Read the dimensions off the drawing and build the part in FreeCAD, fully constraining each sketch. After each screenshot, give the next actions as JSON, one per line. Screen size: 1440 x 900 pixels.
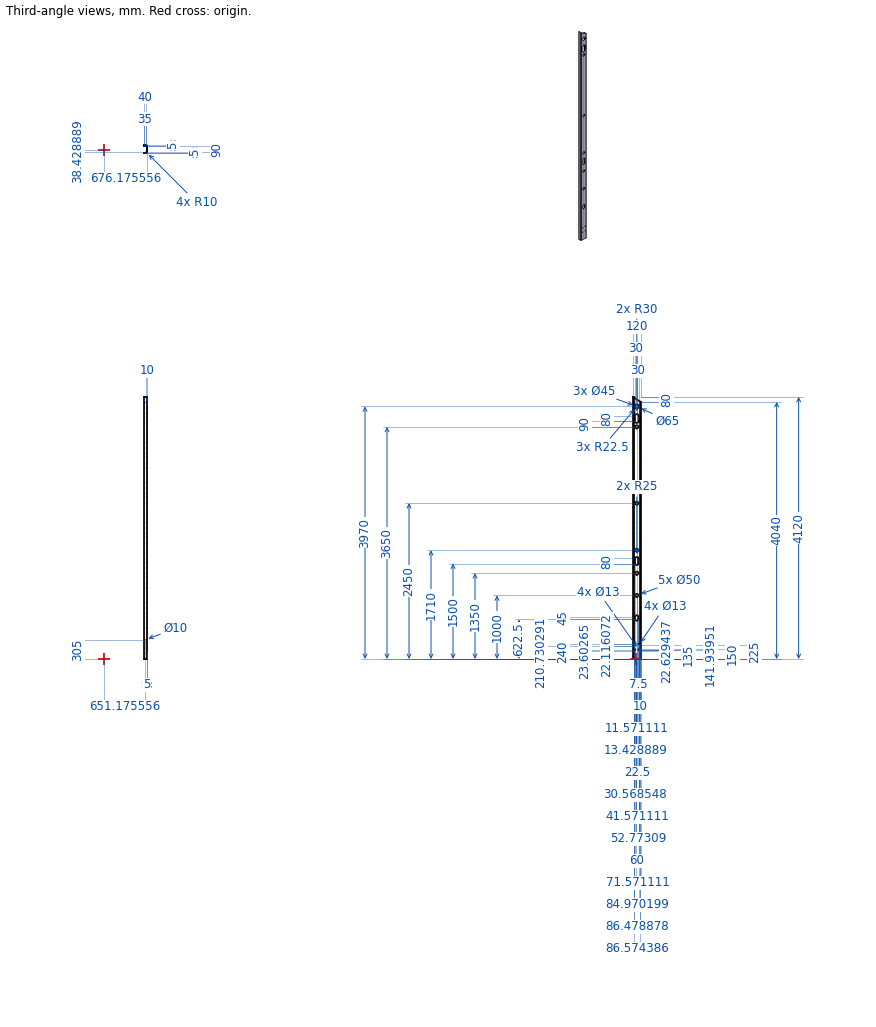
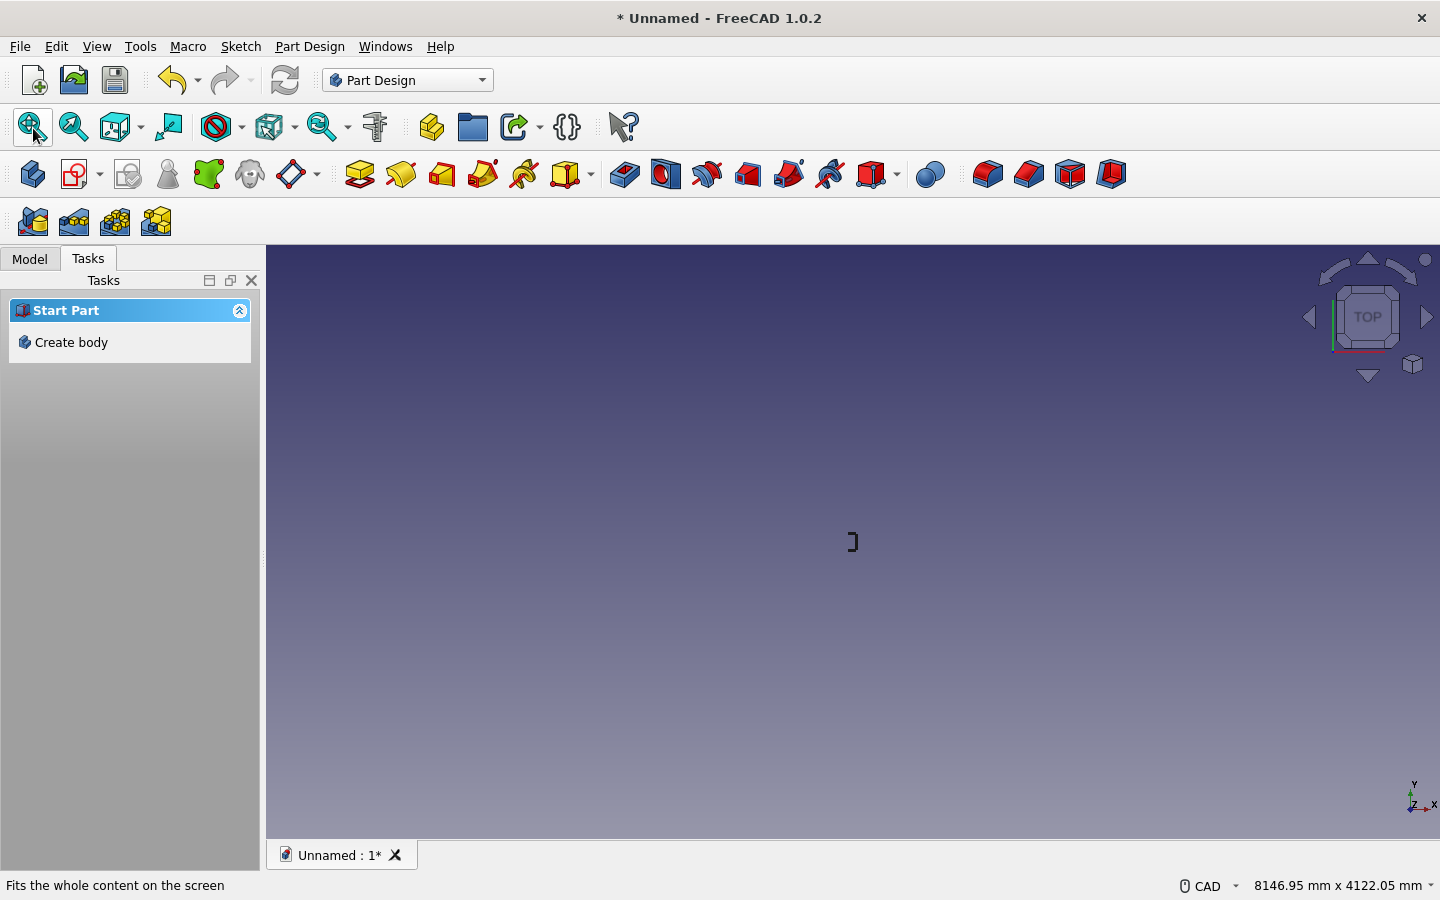
{"action": "key", "text": "v f"}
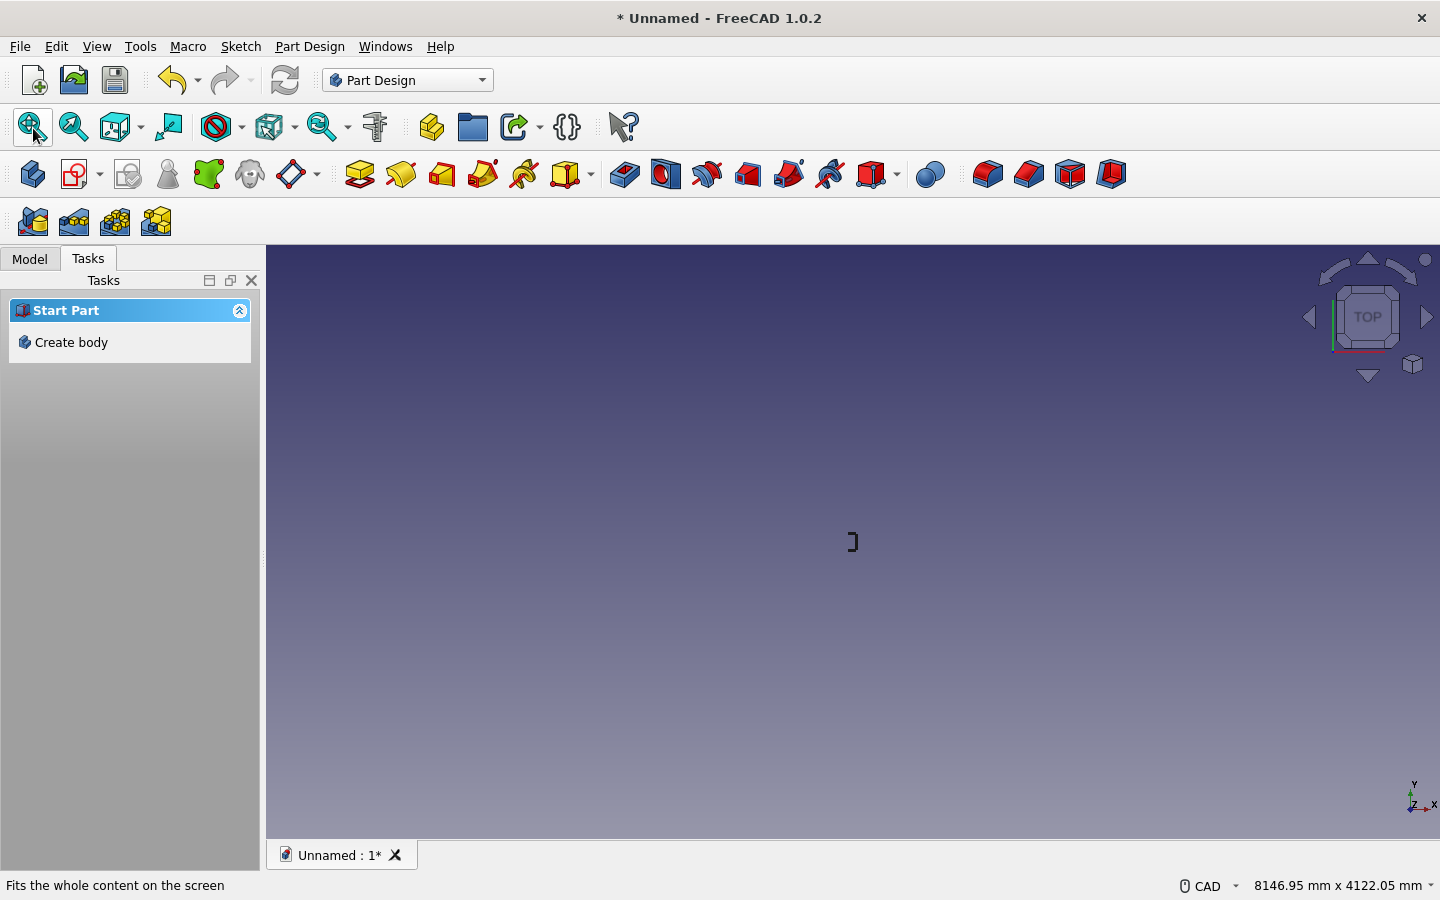
{"action": "left_click", "coordinate": [30, 258]}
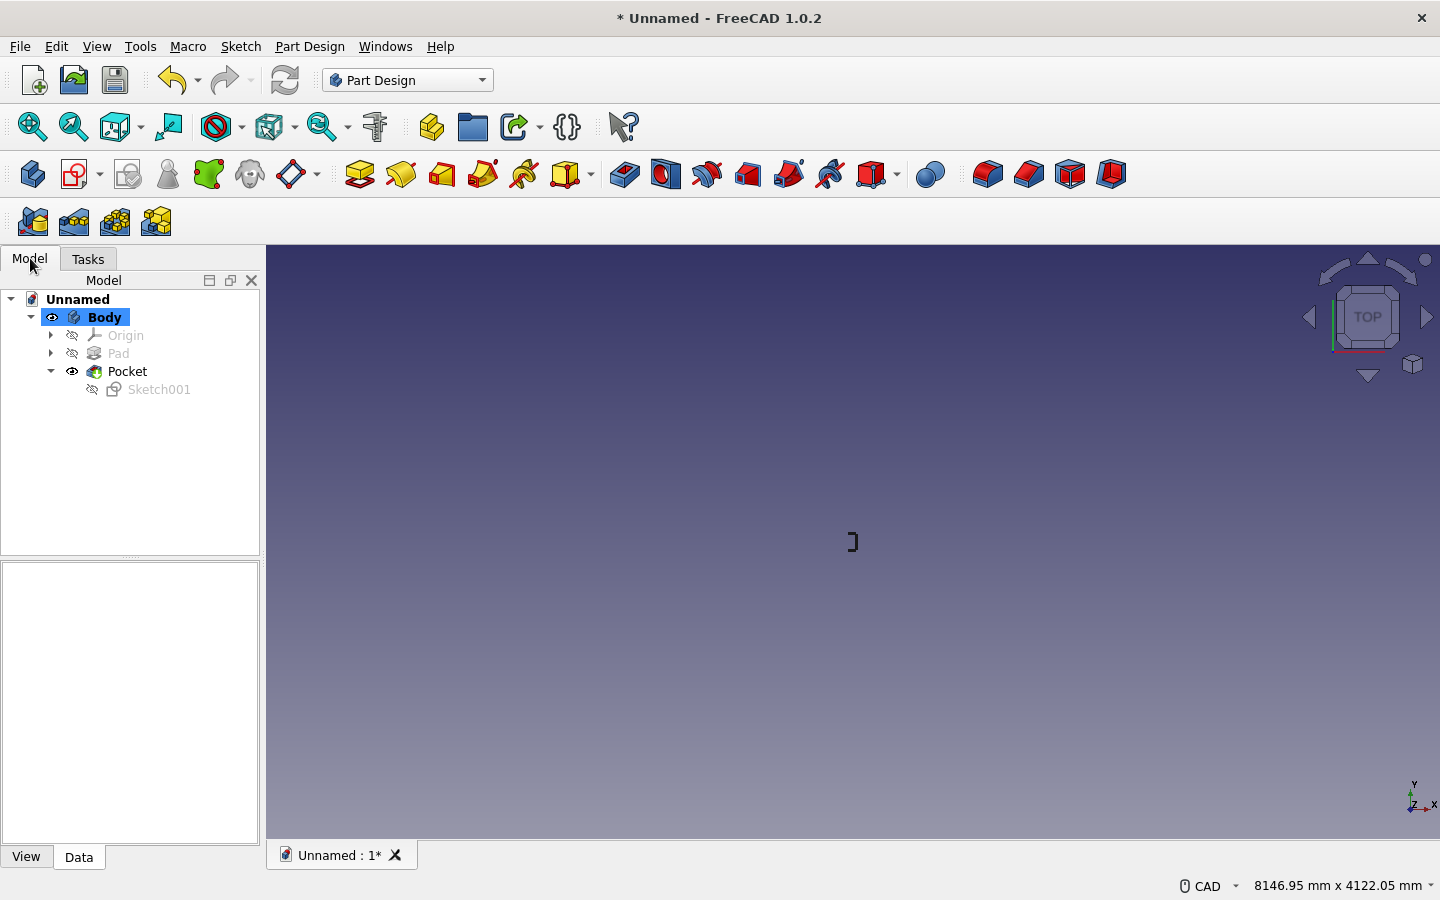
{"action": "left_click", "coordinate": [51, 335]}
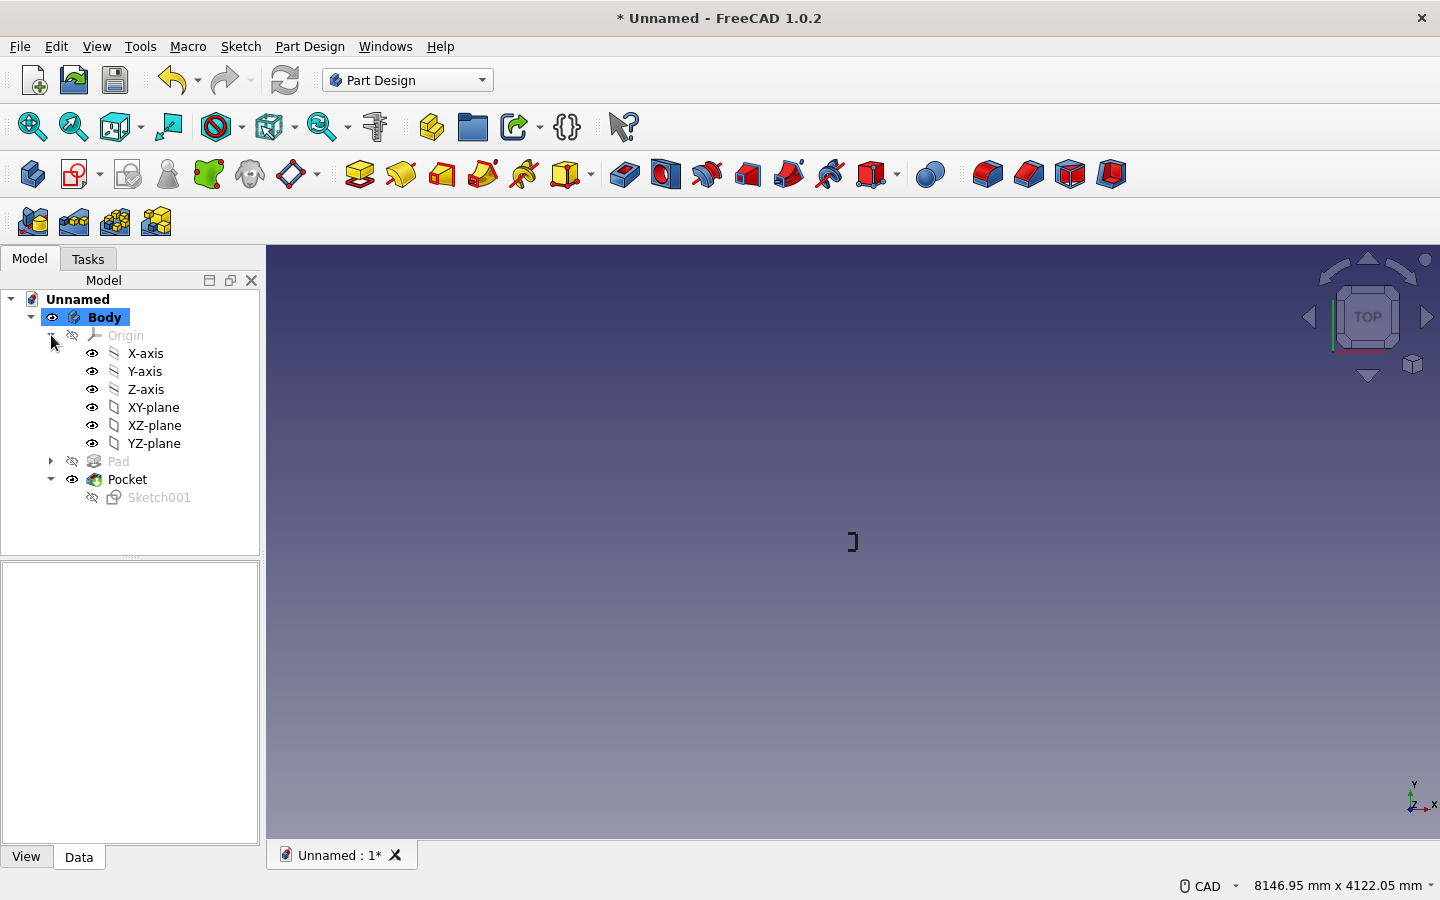
{"action": "left_click", "coordinate": [137, 443]}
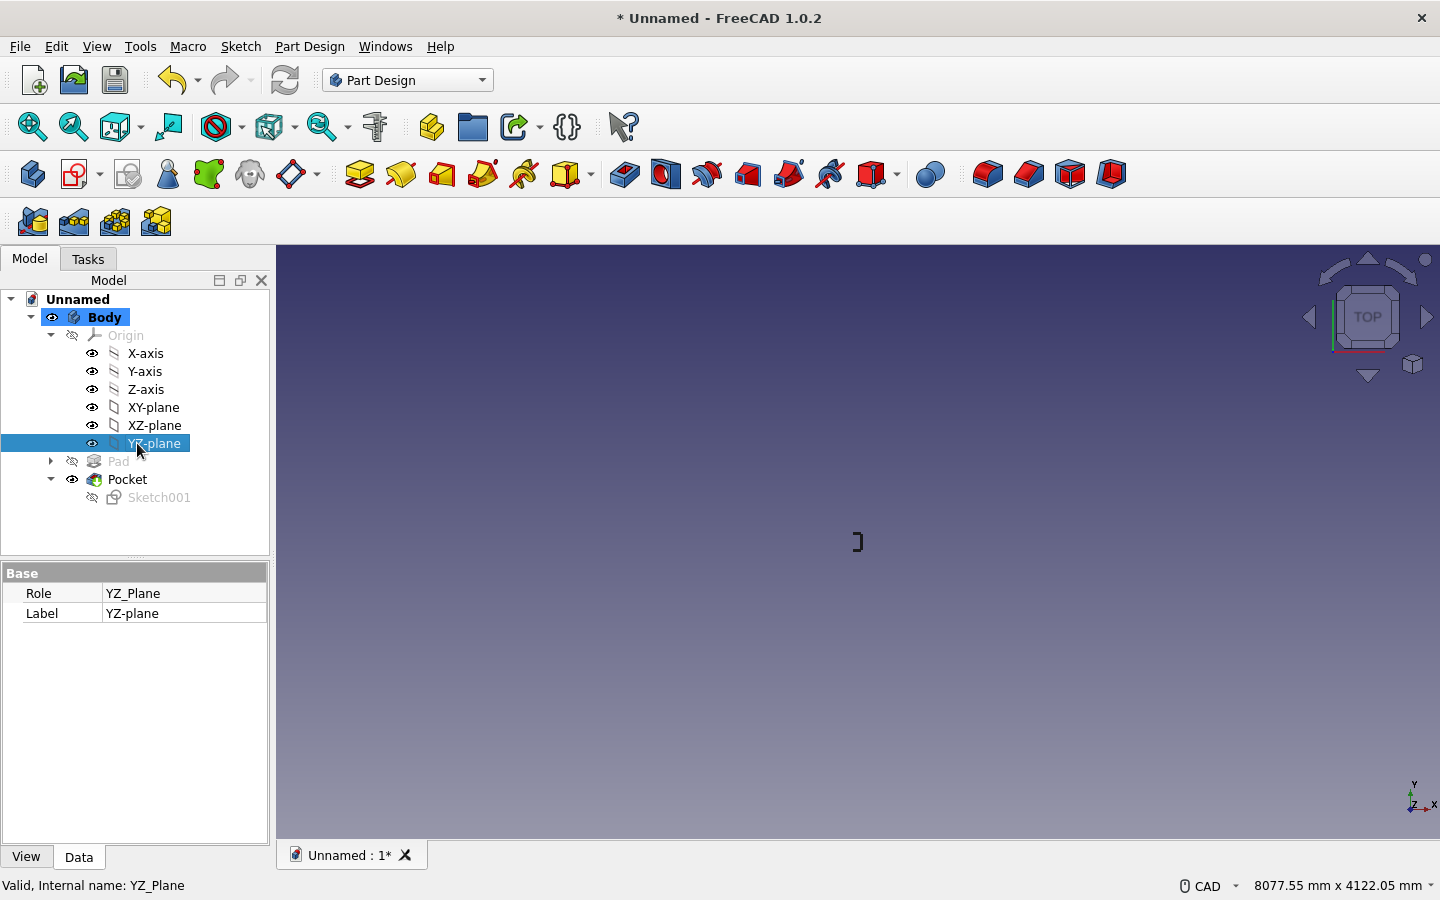
{"action": "left_click", "coordinate": [290, 174]}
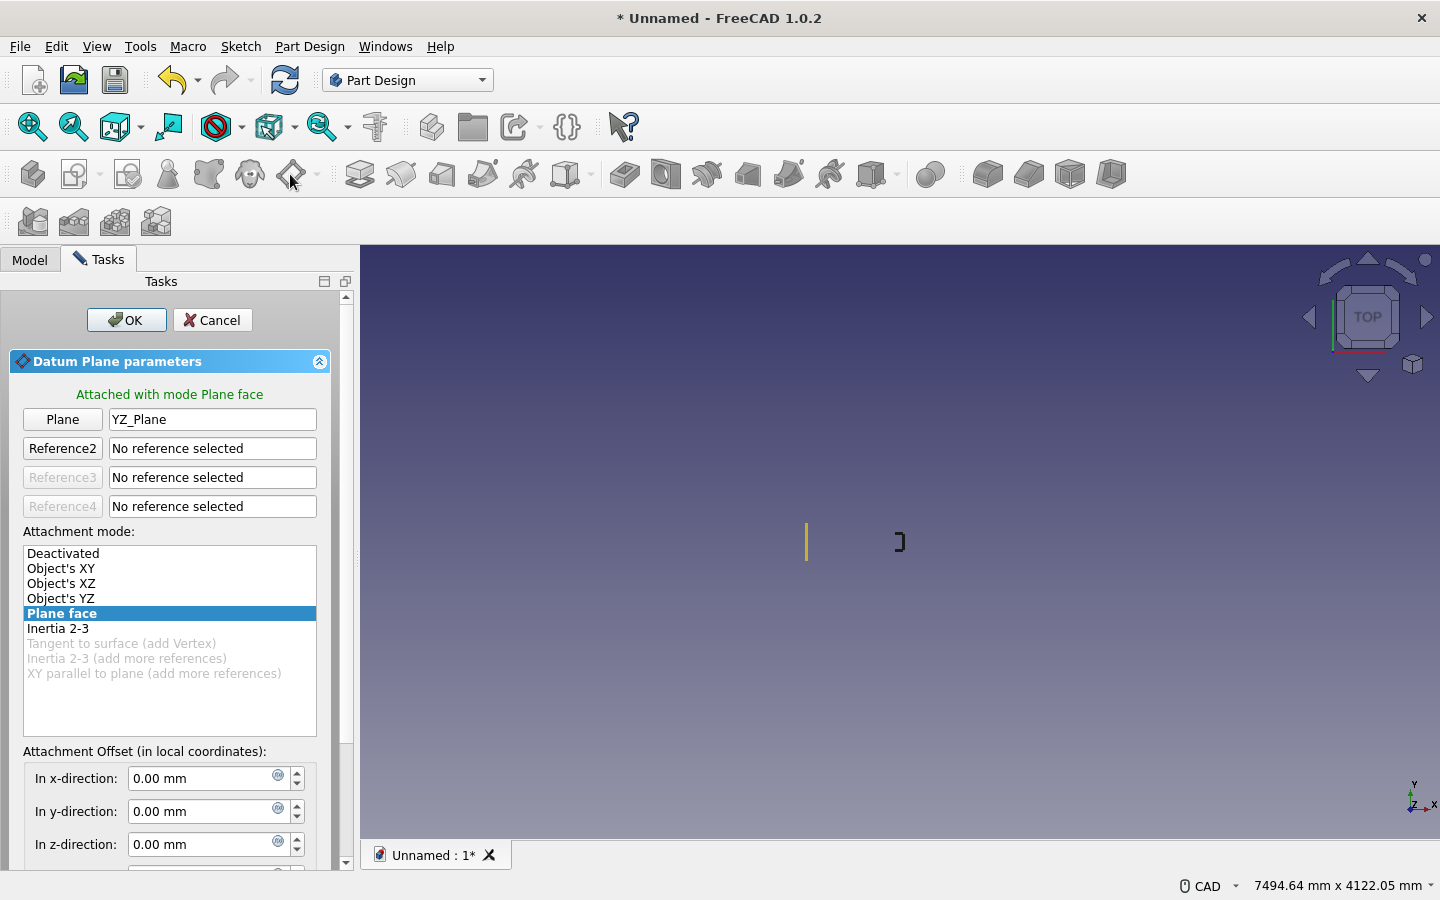
{"action": "triple_click", "coordinate": [210, 844]}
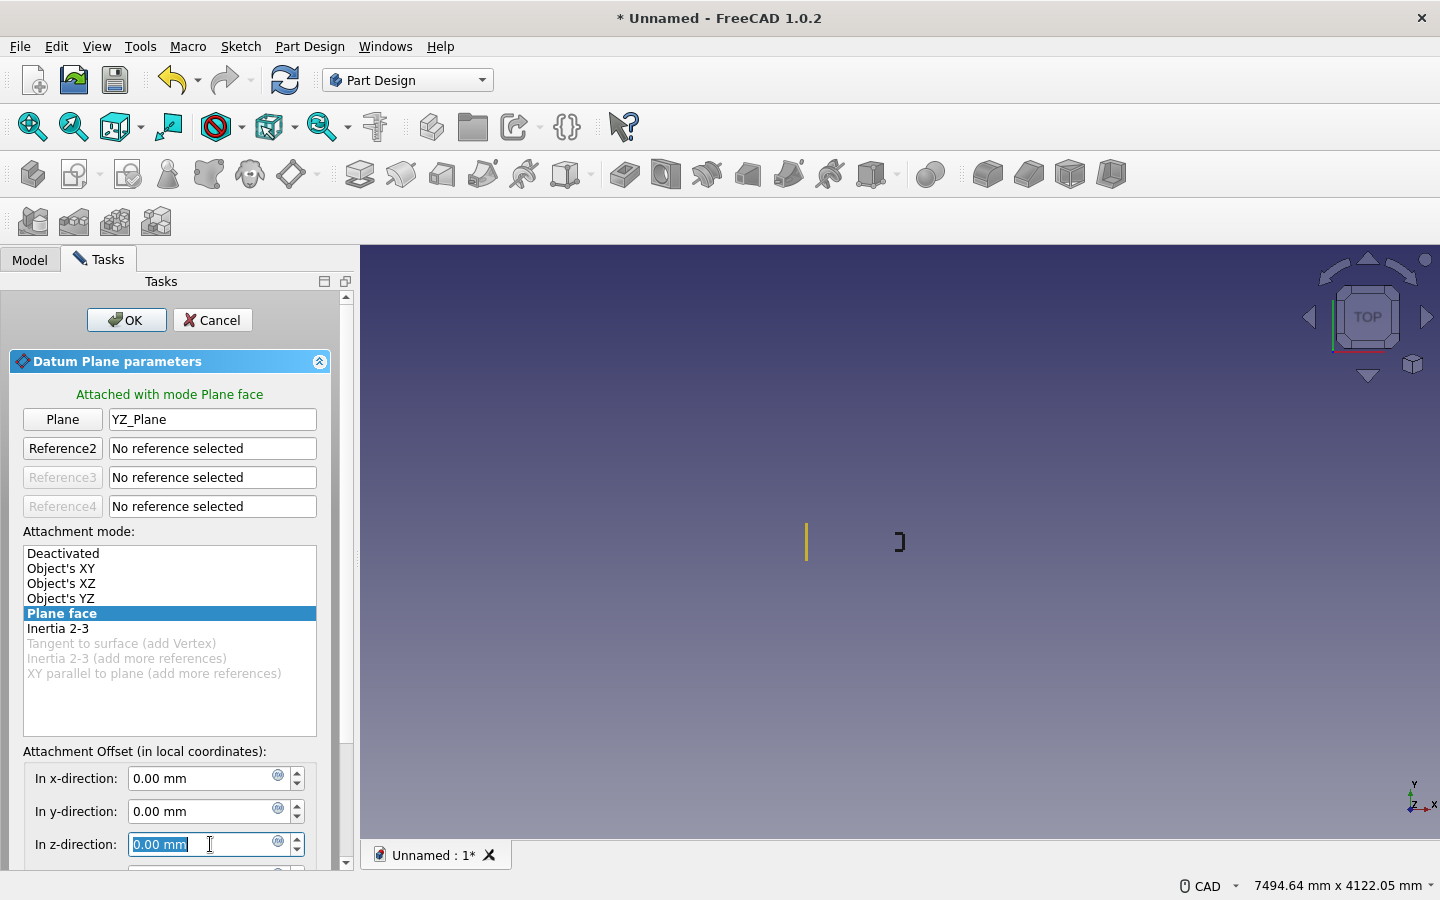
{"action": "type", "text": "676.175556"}
{"action": "key", "text": "Tab"}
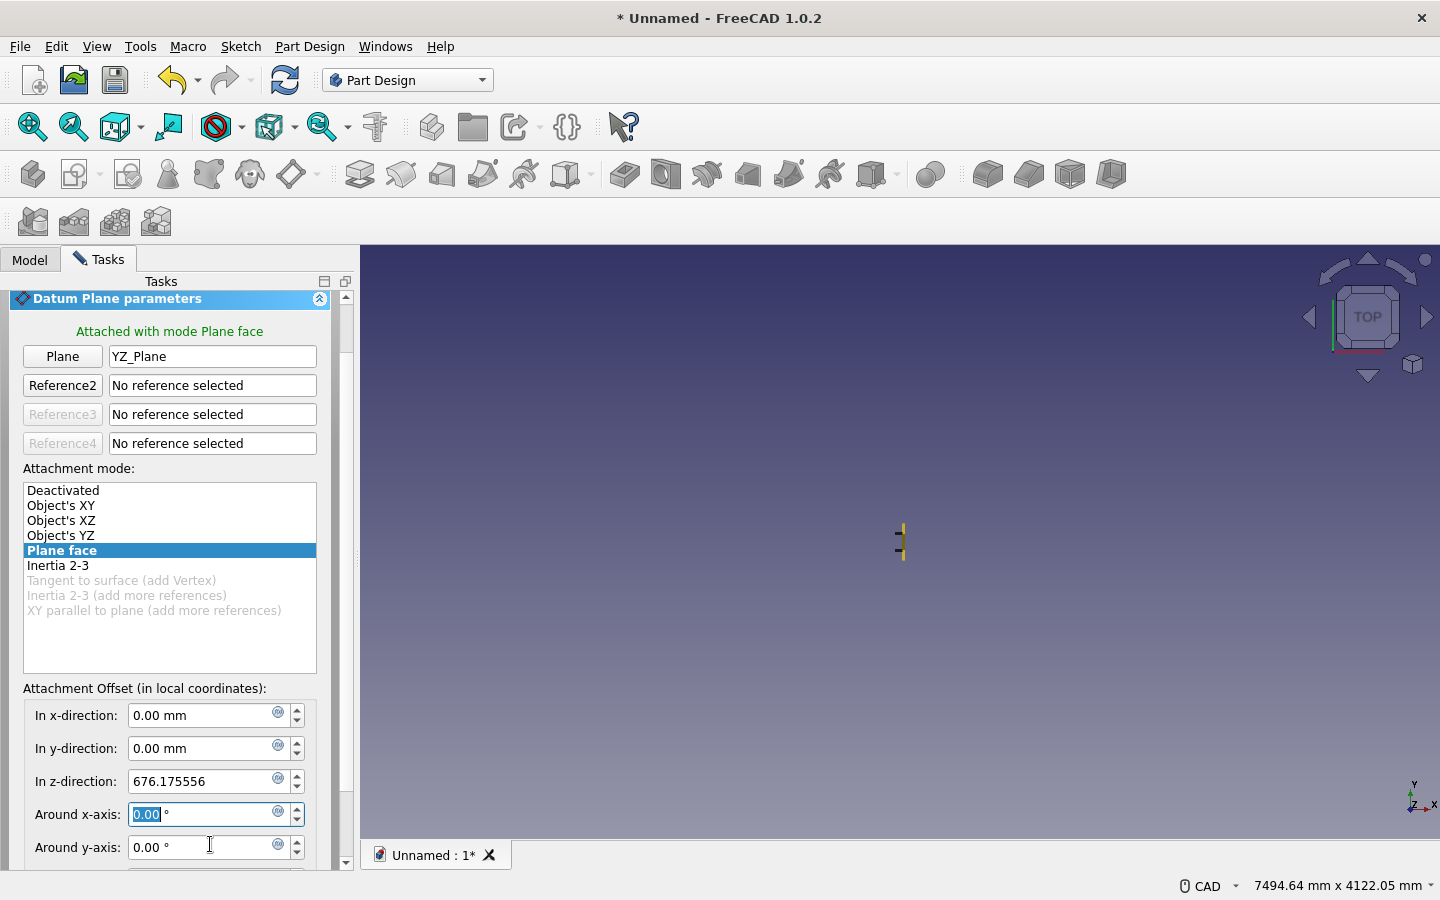
{"action": "scroll", "coordinate": [346, 580], "scroll_direction": "up", "scroll_amount": 2}